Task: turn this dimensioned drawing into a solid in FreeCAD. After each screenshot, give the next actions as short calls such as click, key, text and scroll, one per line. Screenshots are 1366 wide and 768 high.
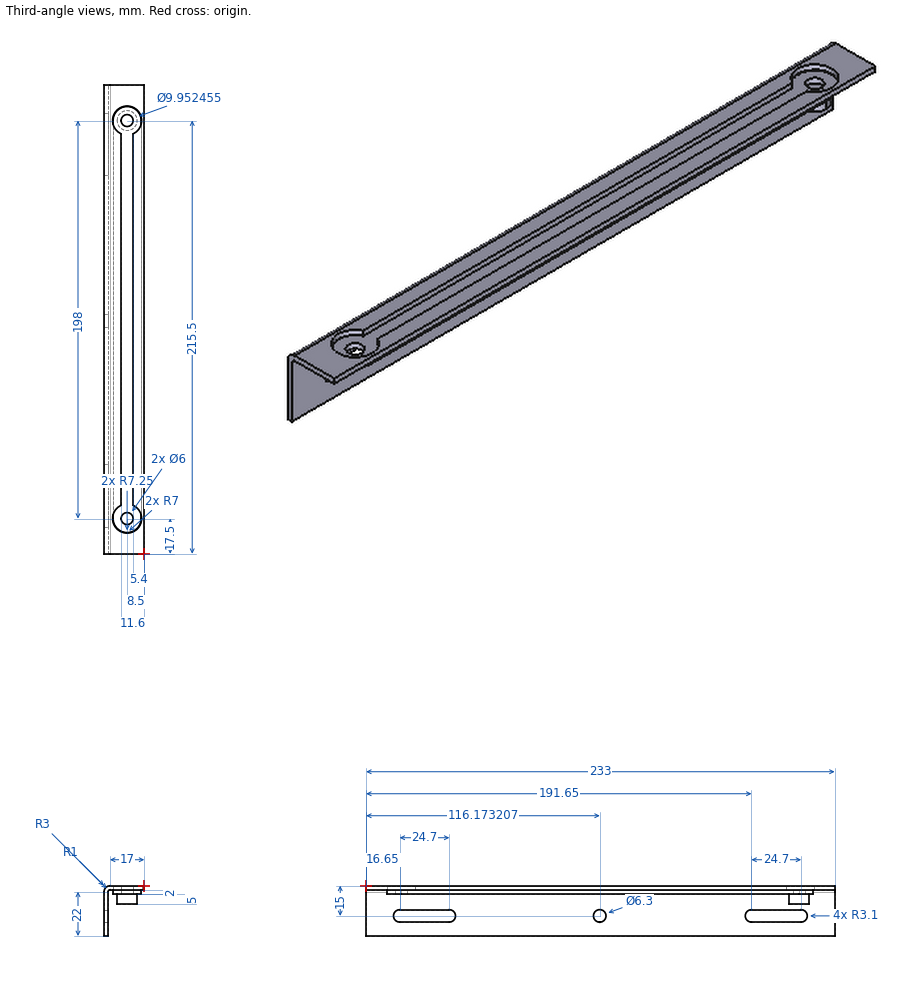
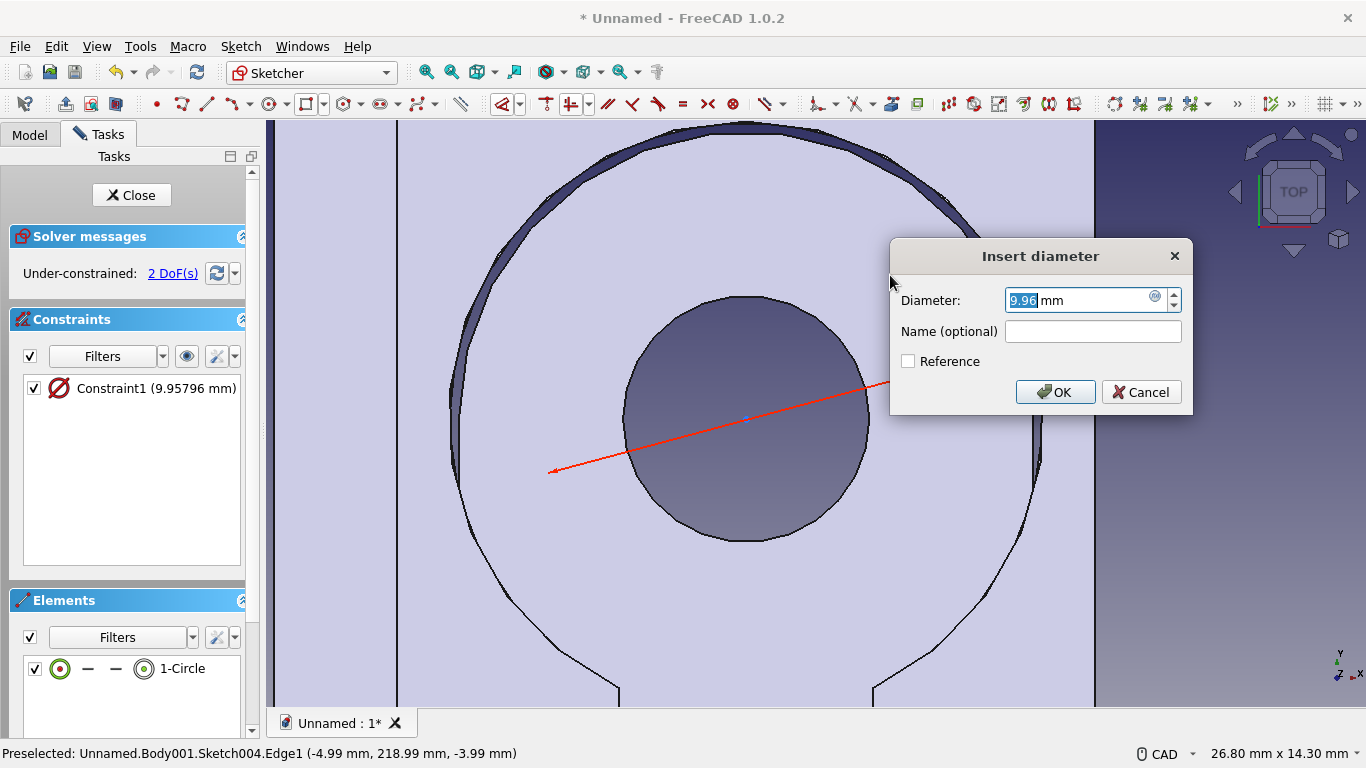
text(9.952455)
key(Return)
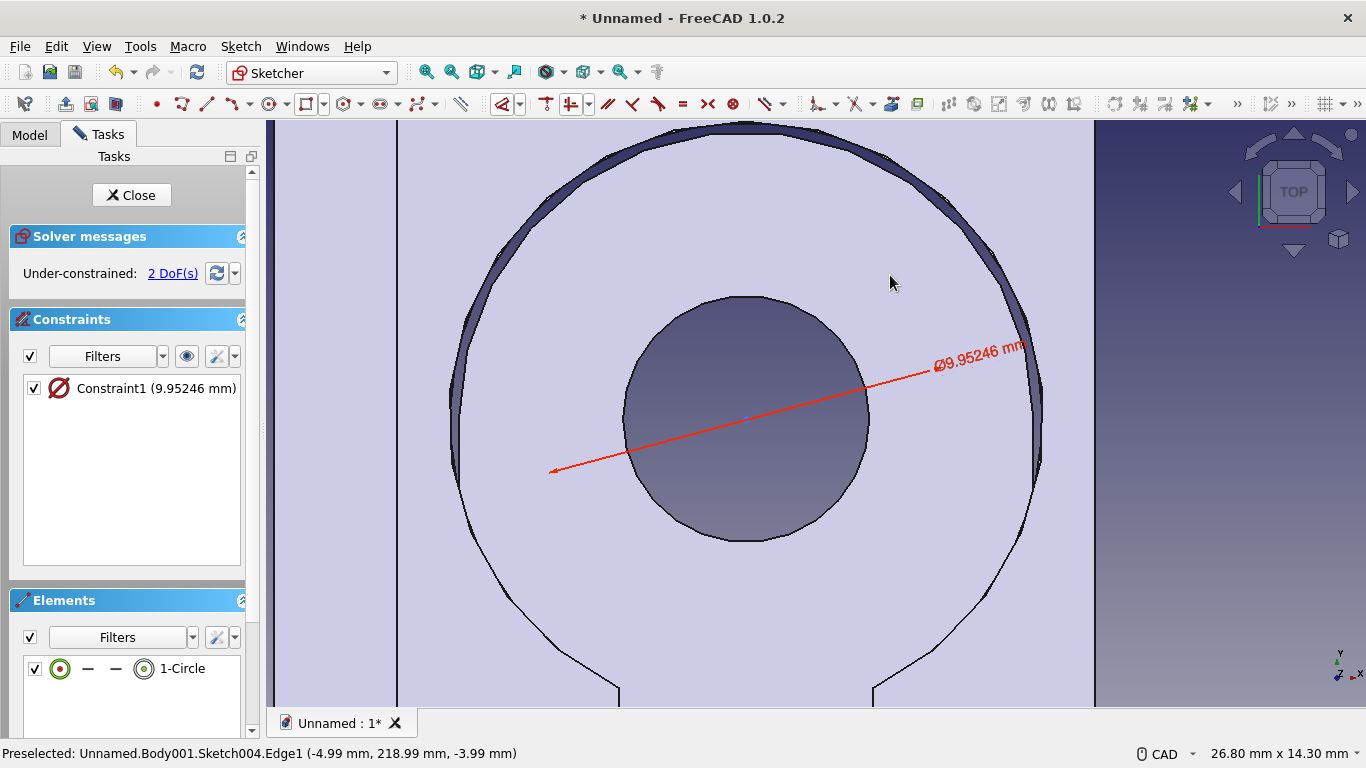
click(746, 420)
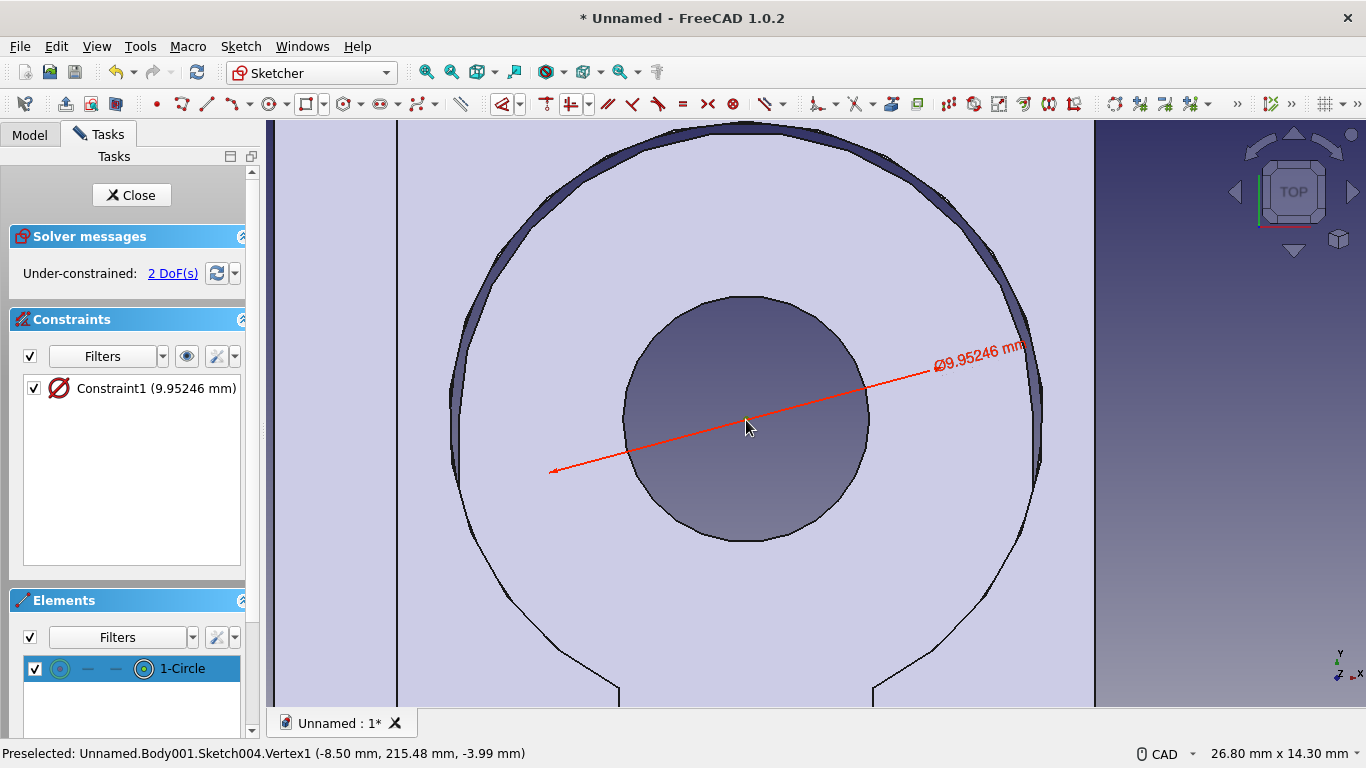
click(520, 104)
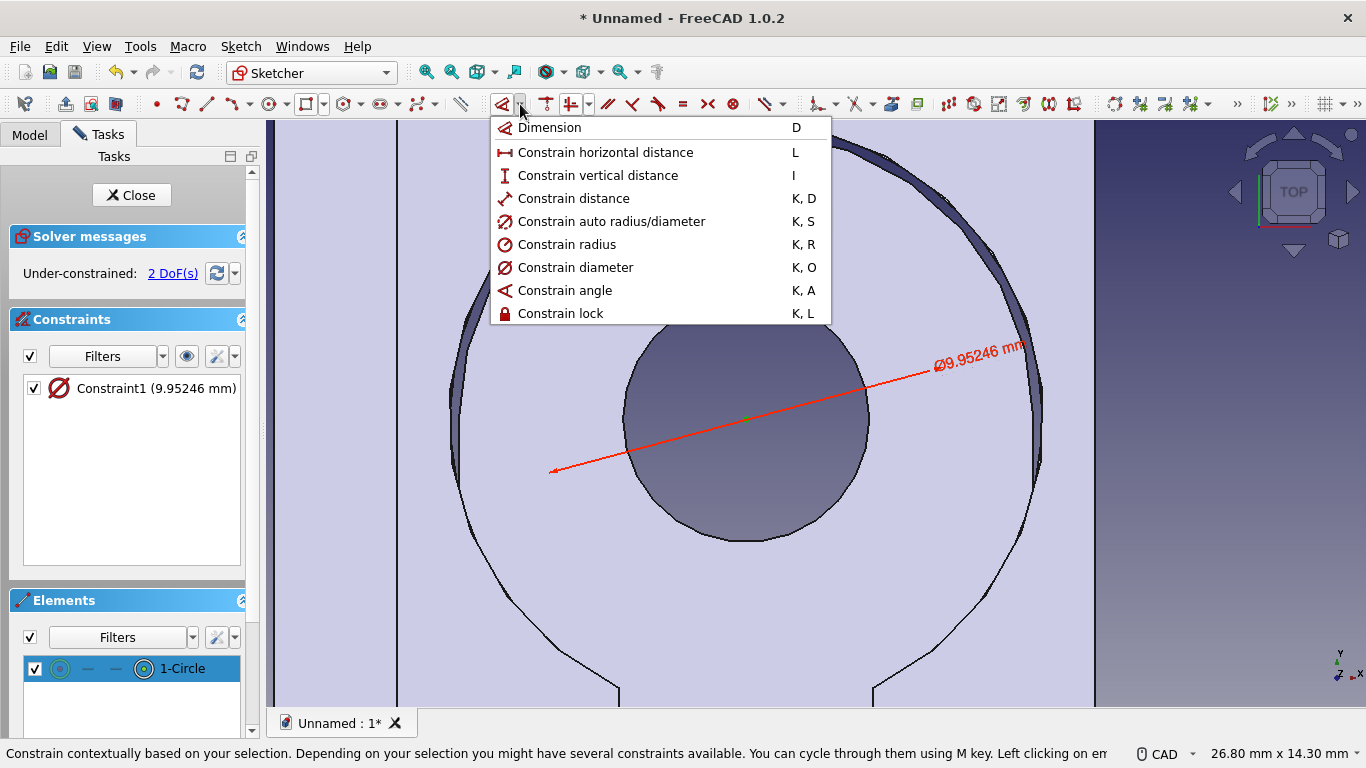
click(661, 152)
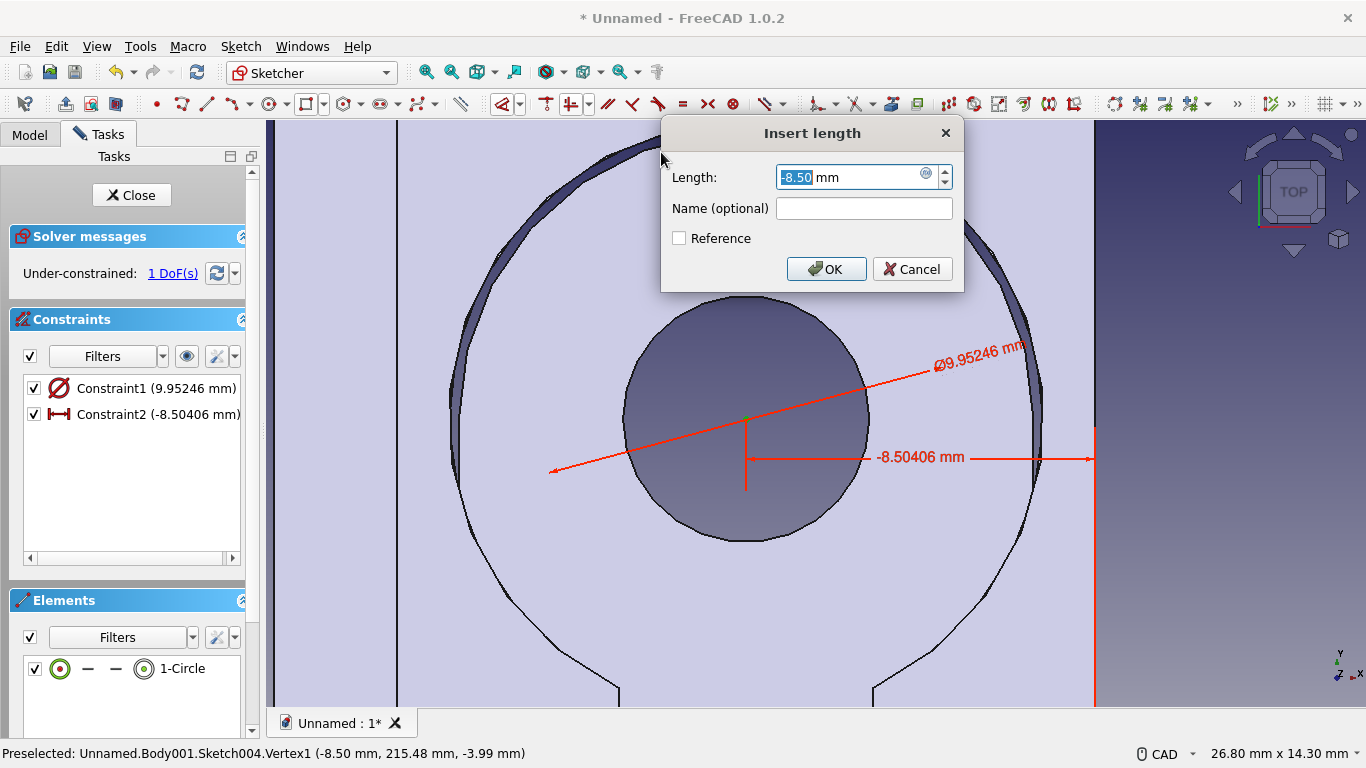
text(-8.5)
key(Return)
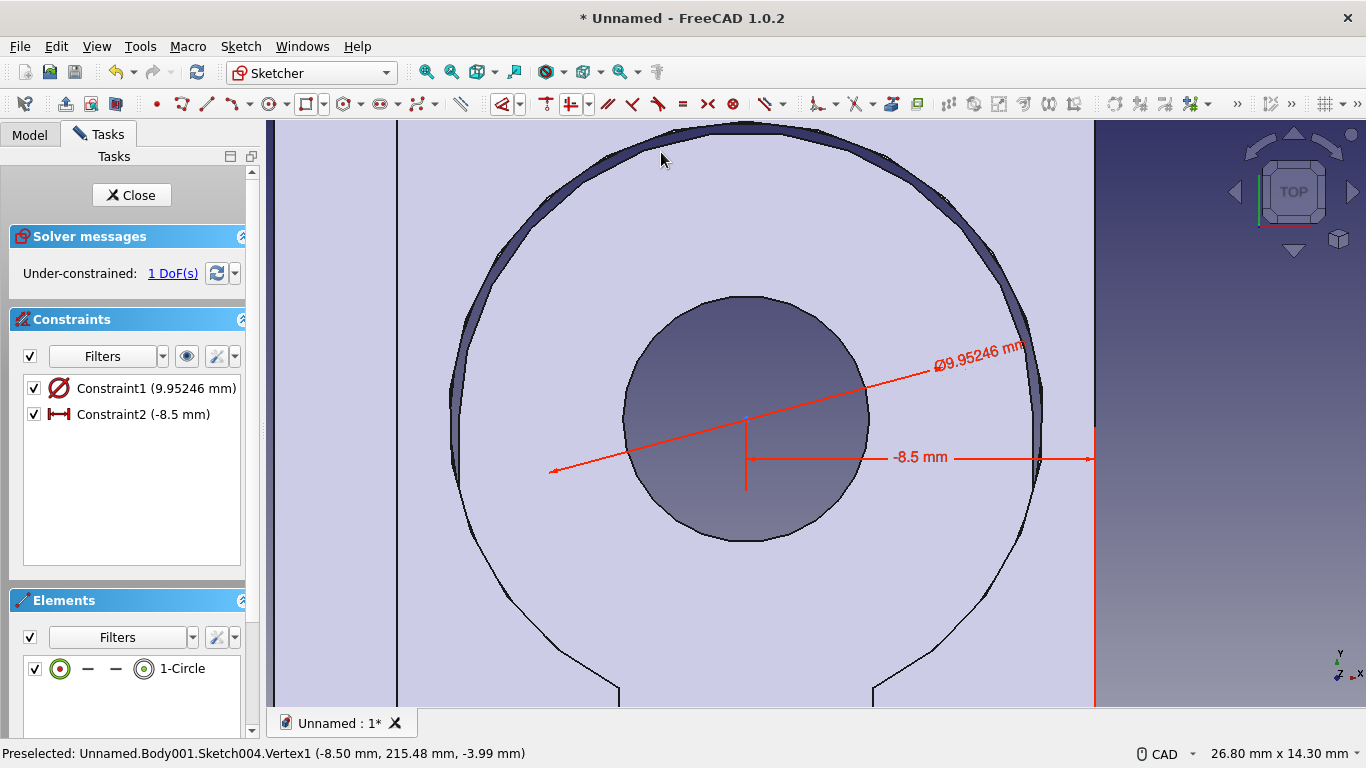
click(746, 420)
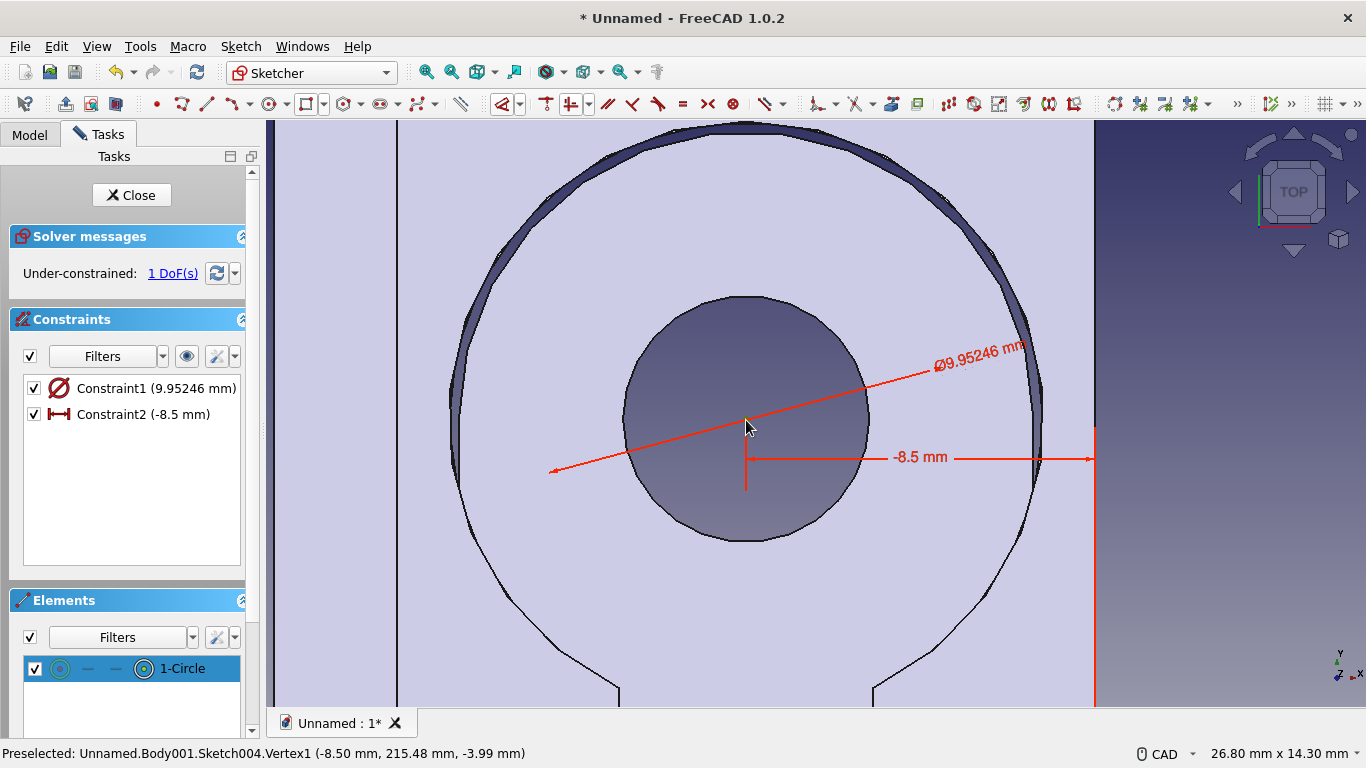
click(520, 104)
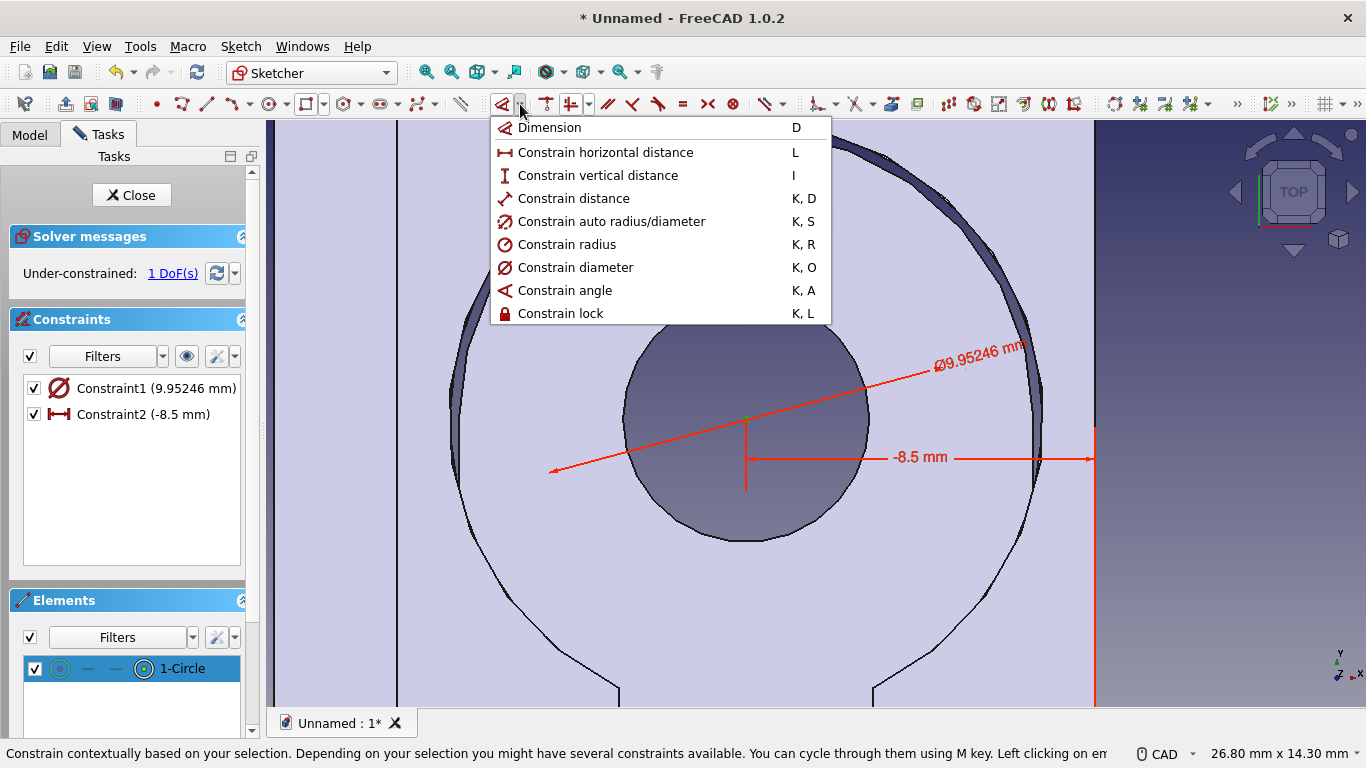
click(661, 176)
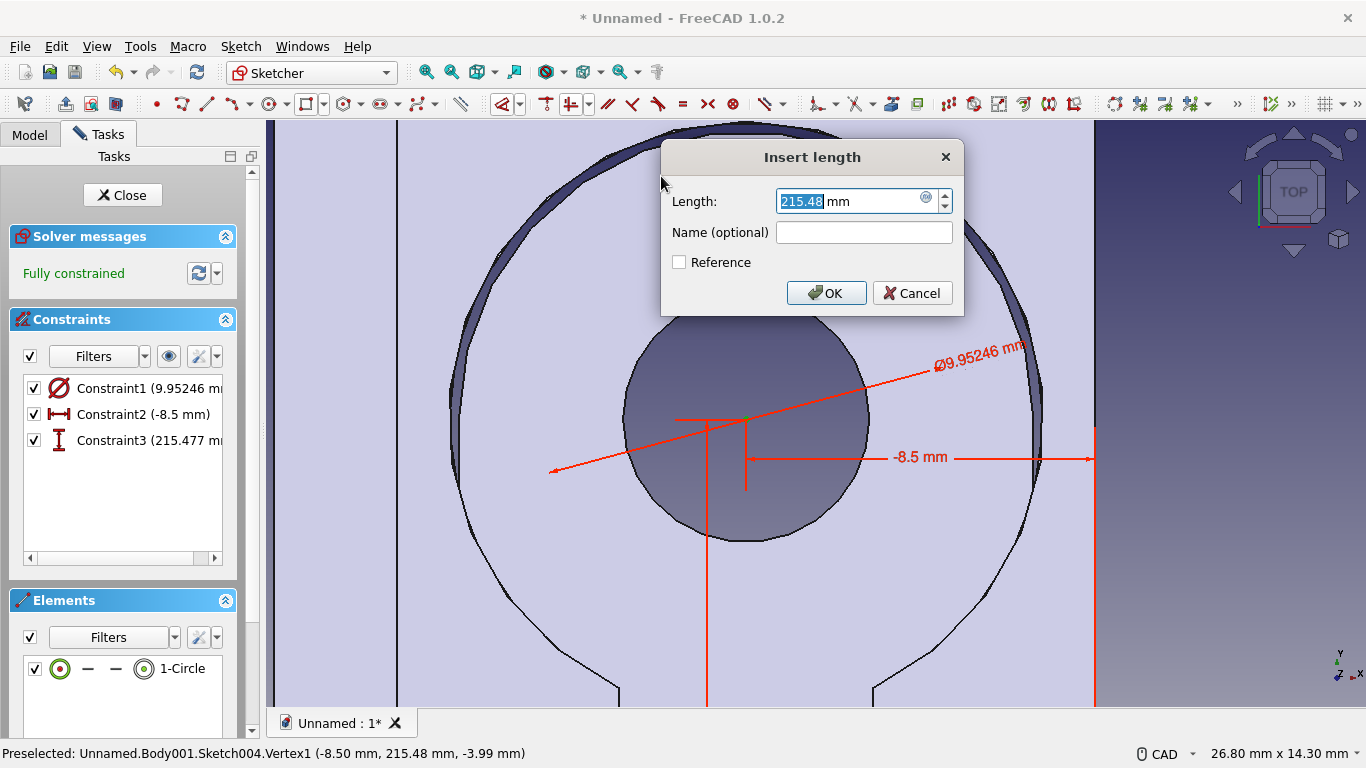
text(215.5)
key(Return)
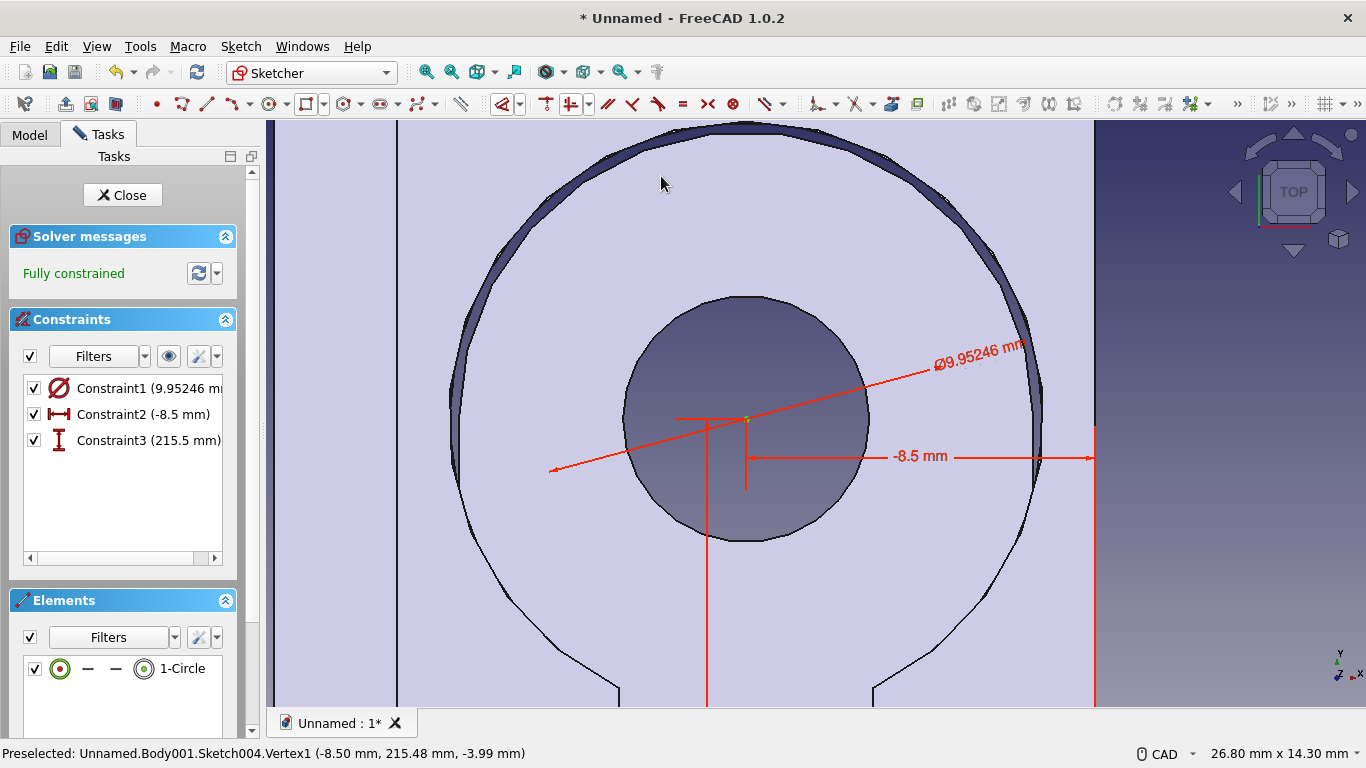
click(123, 195)